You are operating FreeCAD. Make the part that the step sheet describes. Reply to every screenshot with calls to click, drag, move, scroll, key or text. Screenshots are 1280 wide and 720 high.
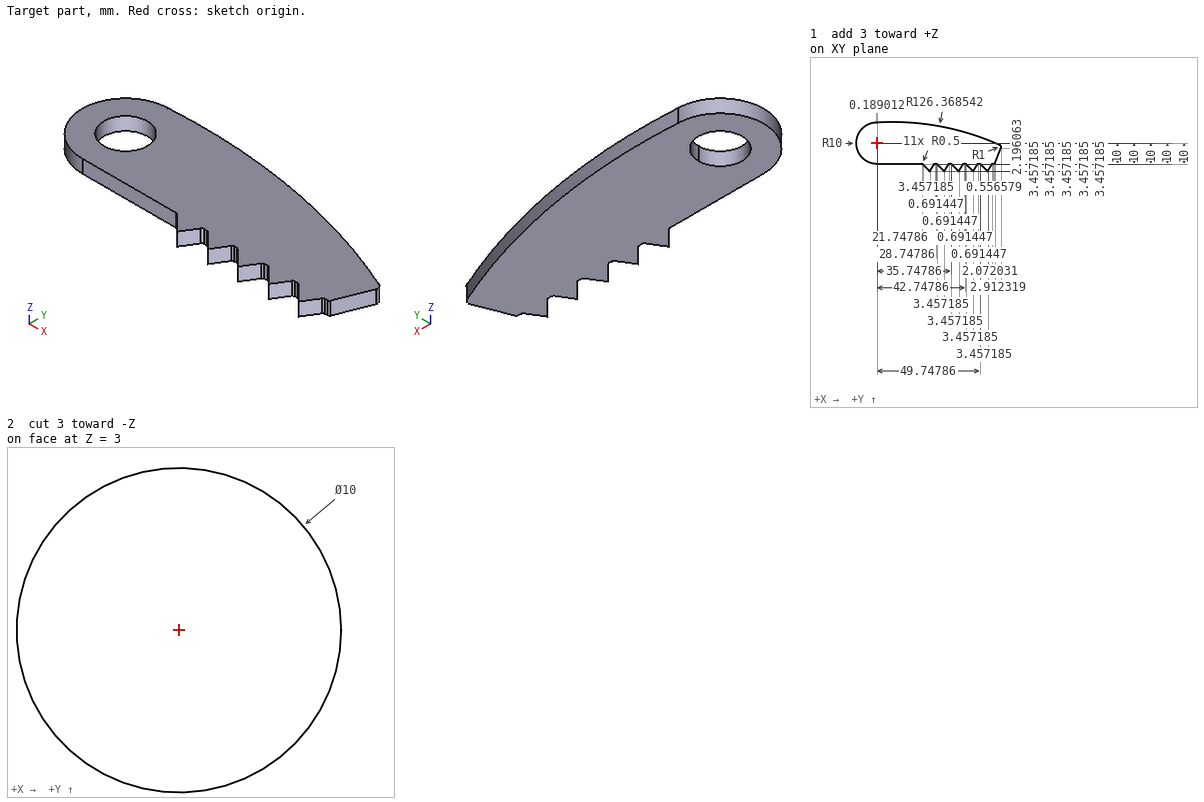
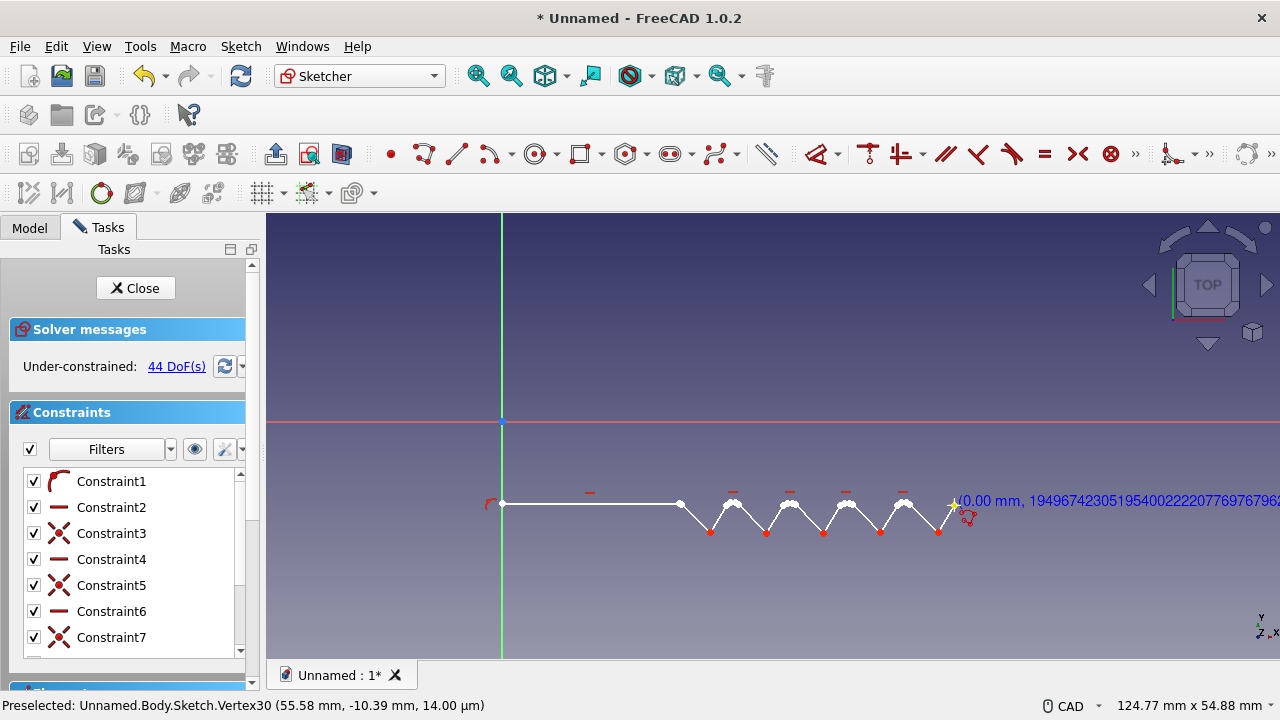
key(g)
key(l)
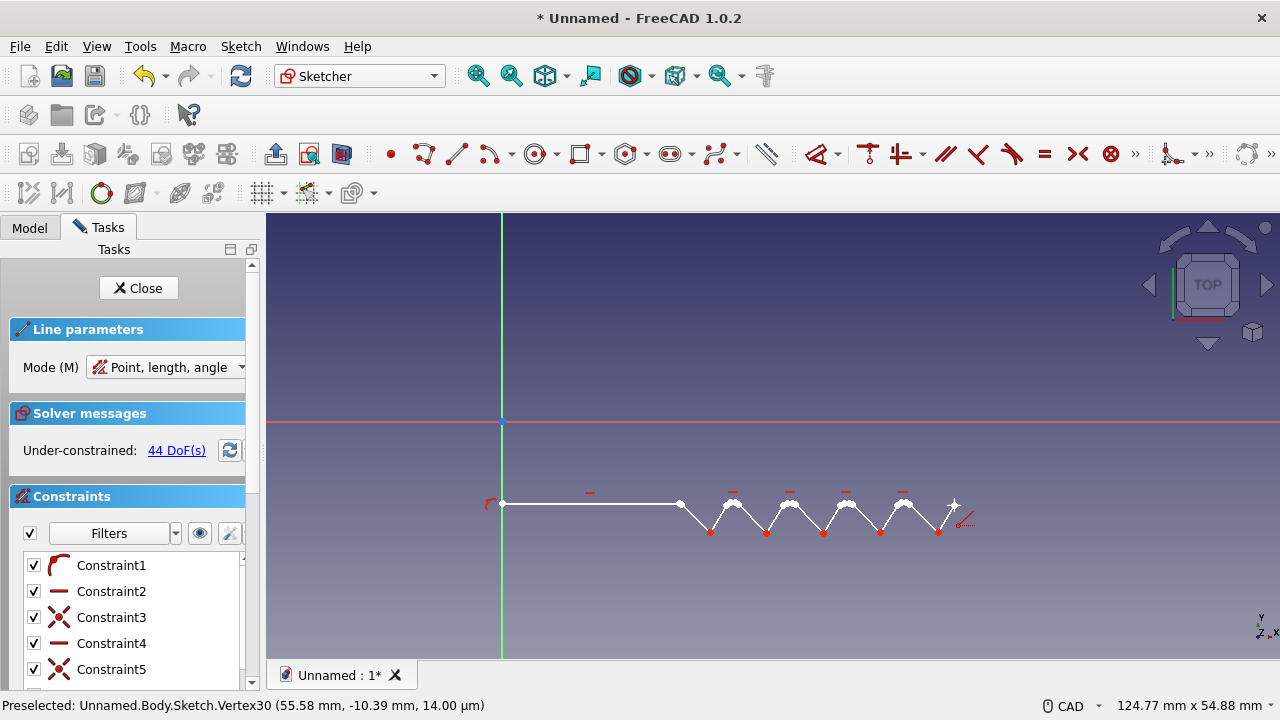
scroll(958, 503, up, 7)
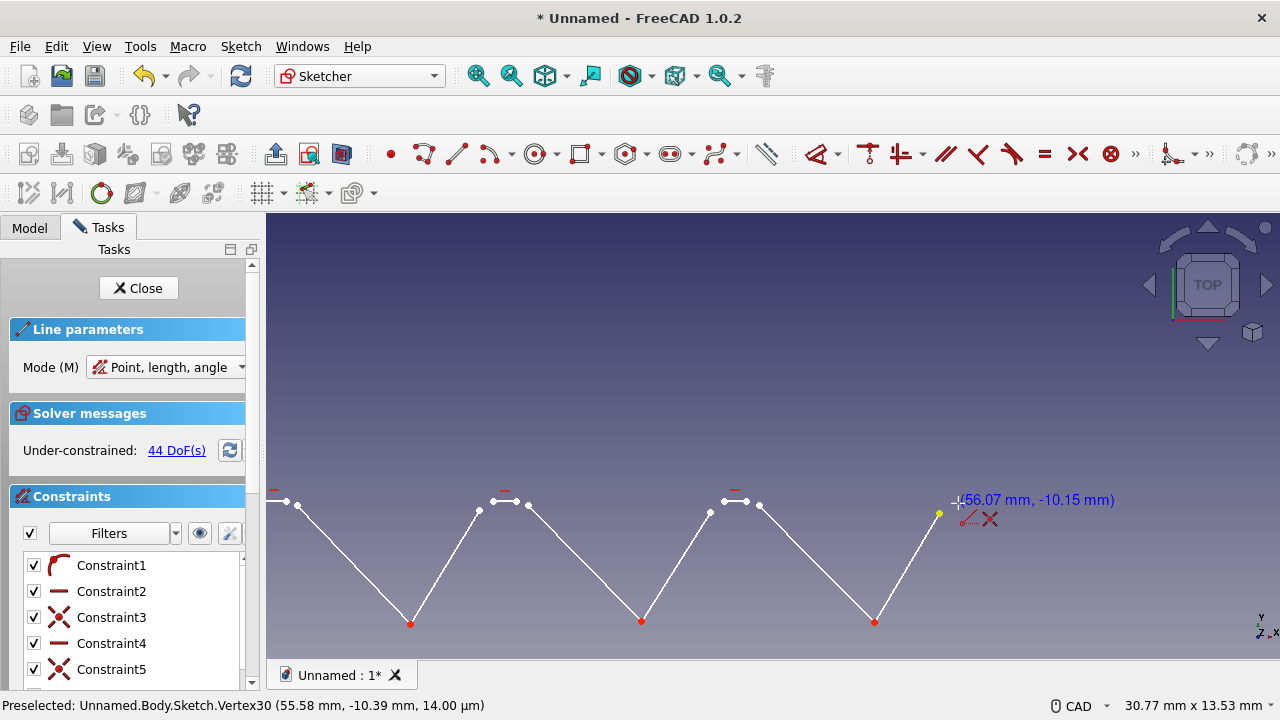
click(955, 500)
click(974, 500)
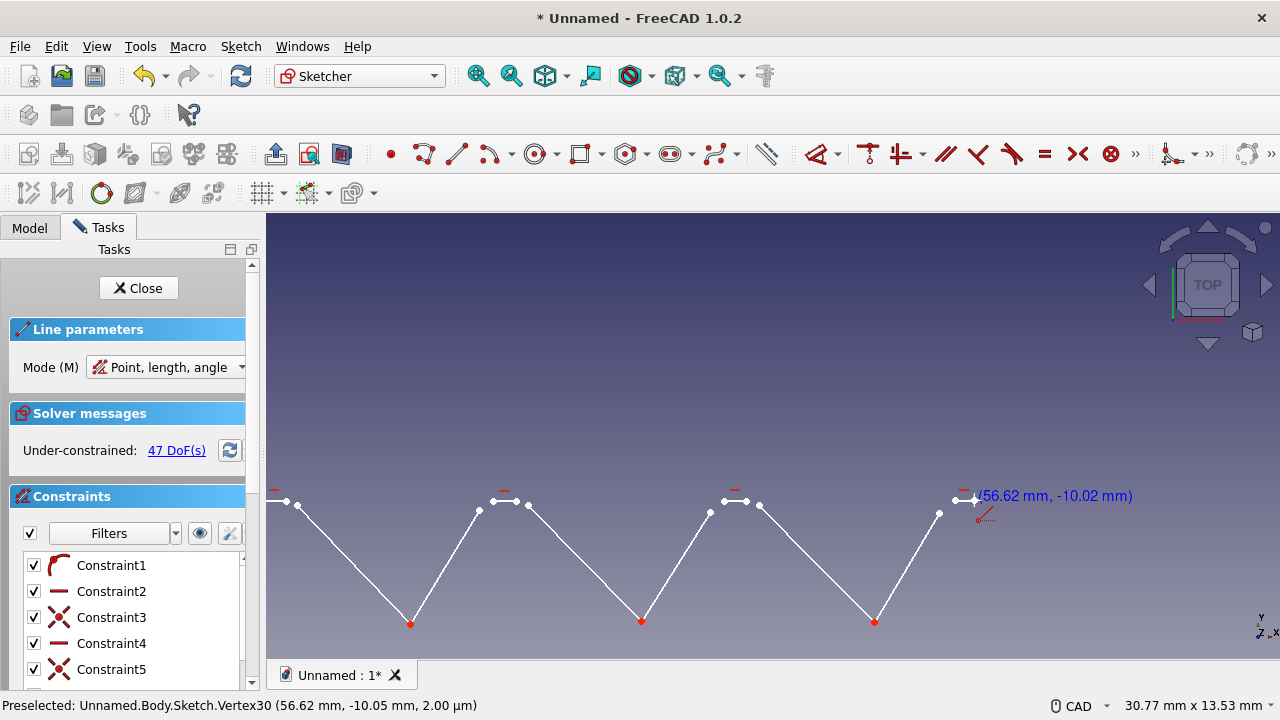
click(989, 490)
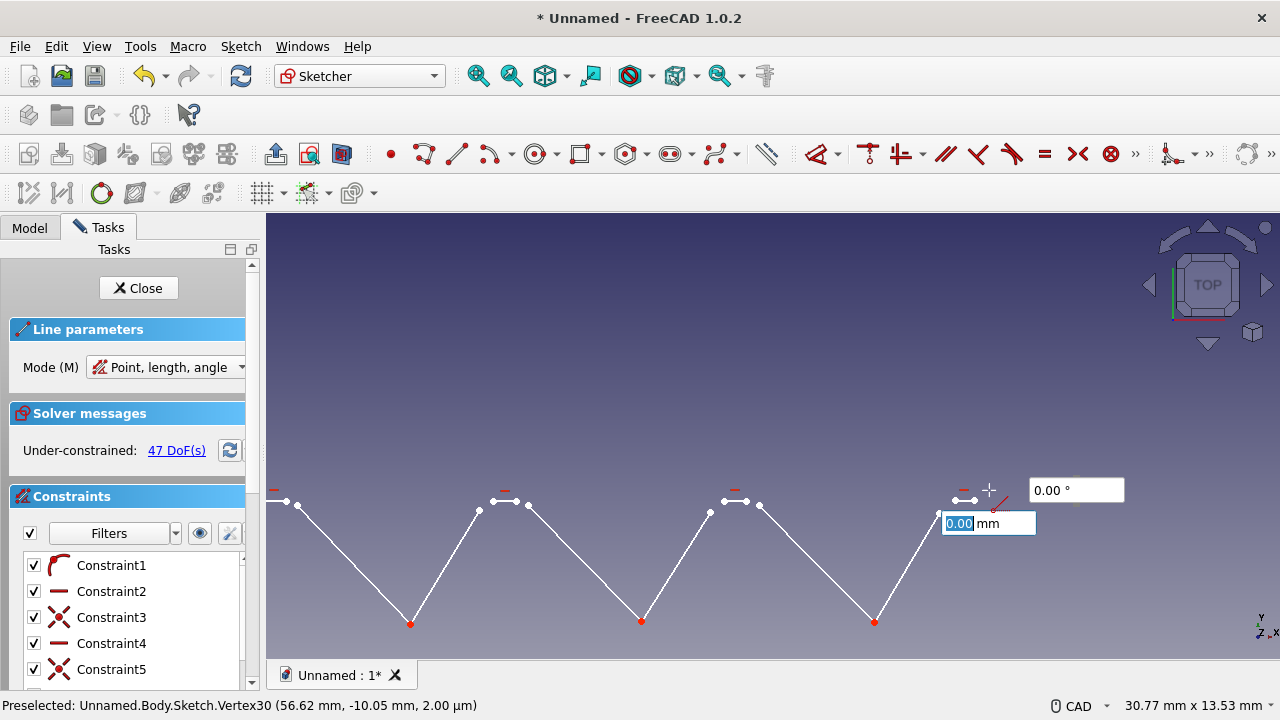
scroll(957, 503, down, 7)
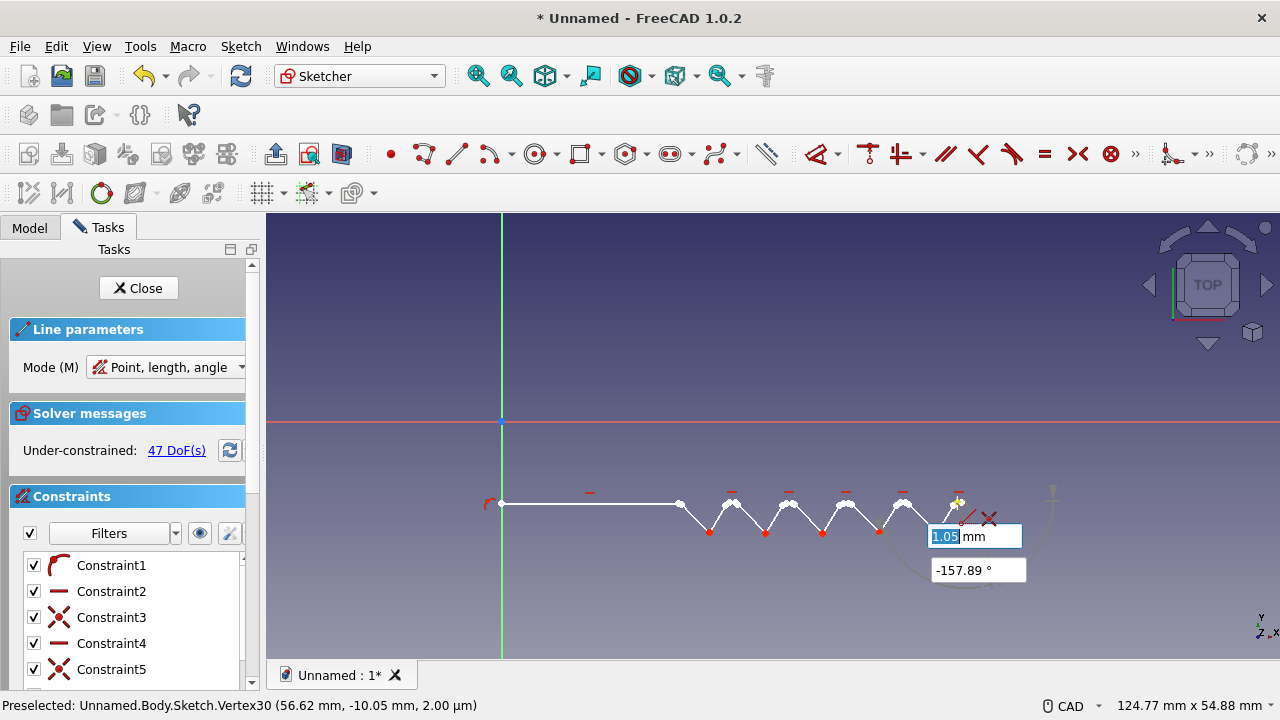
click(989, 439)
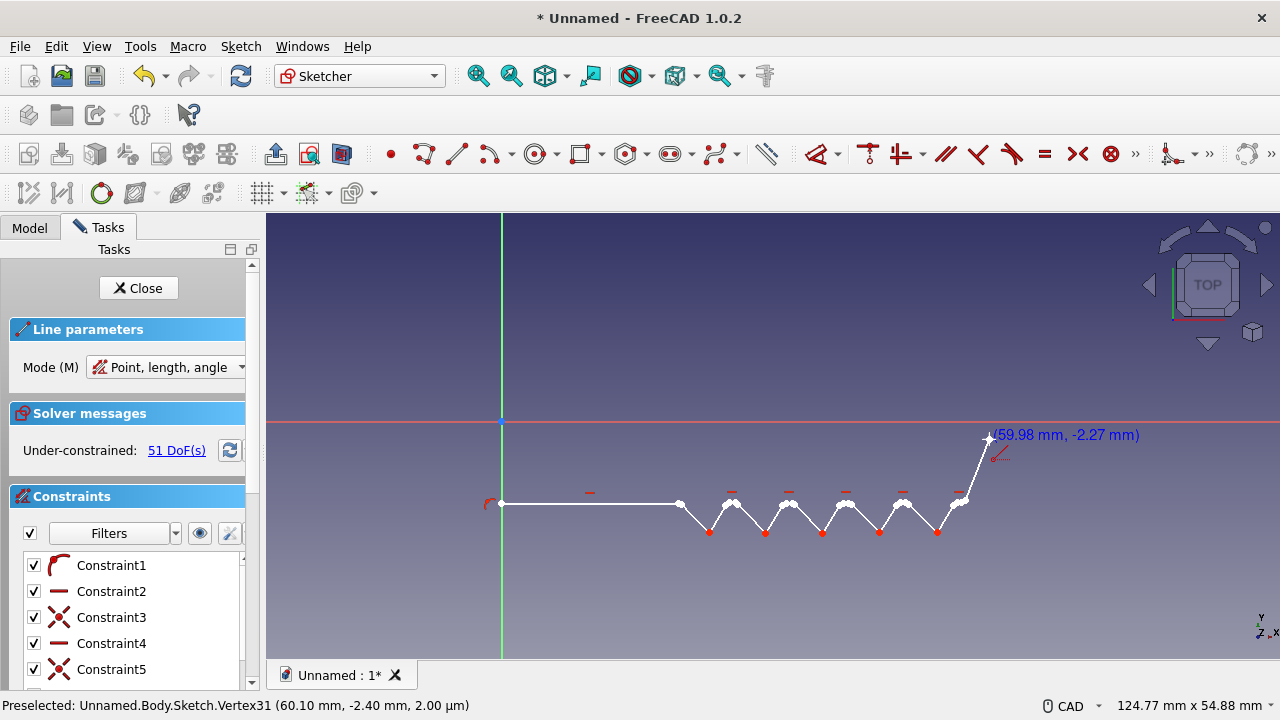
click(512, 154)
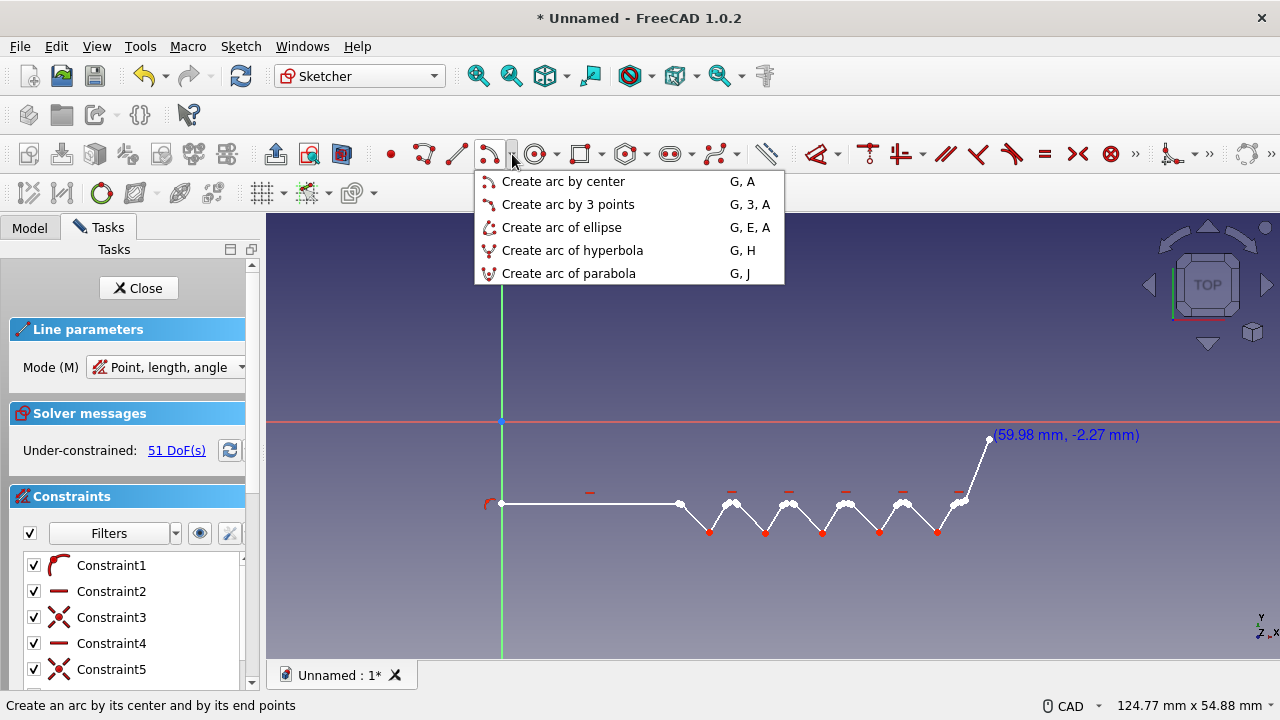
click(630, 204)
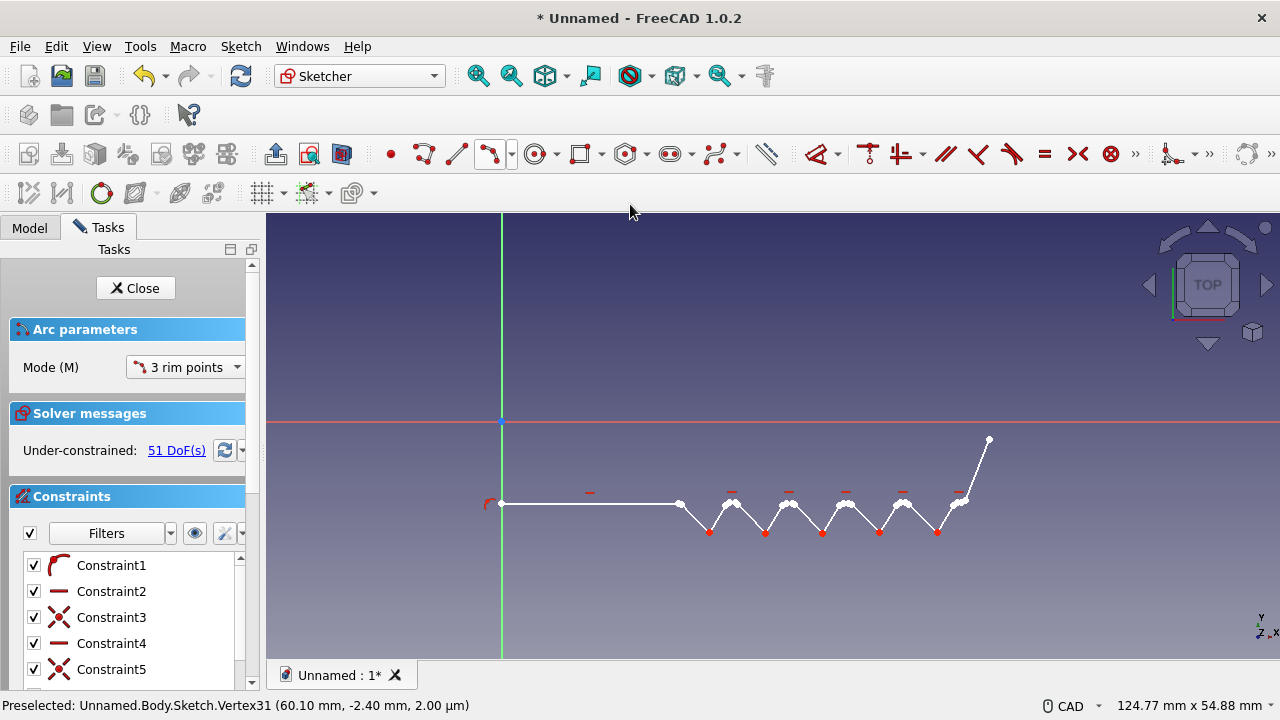
scroll(678, 503, up, 9)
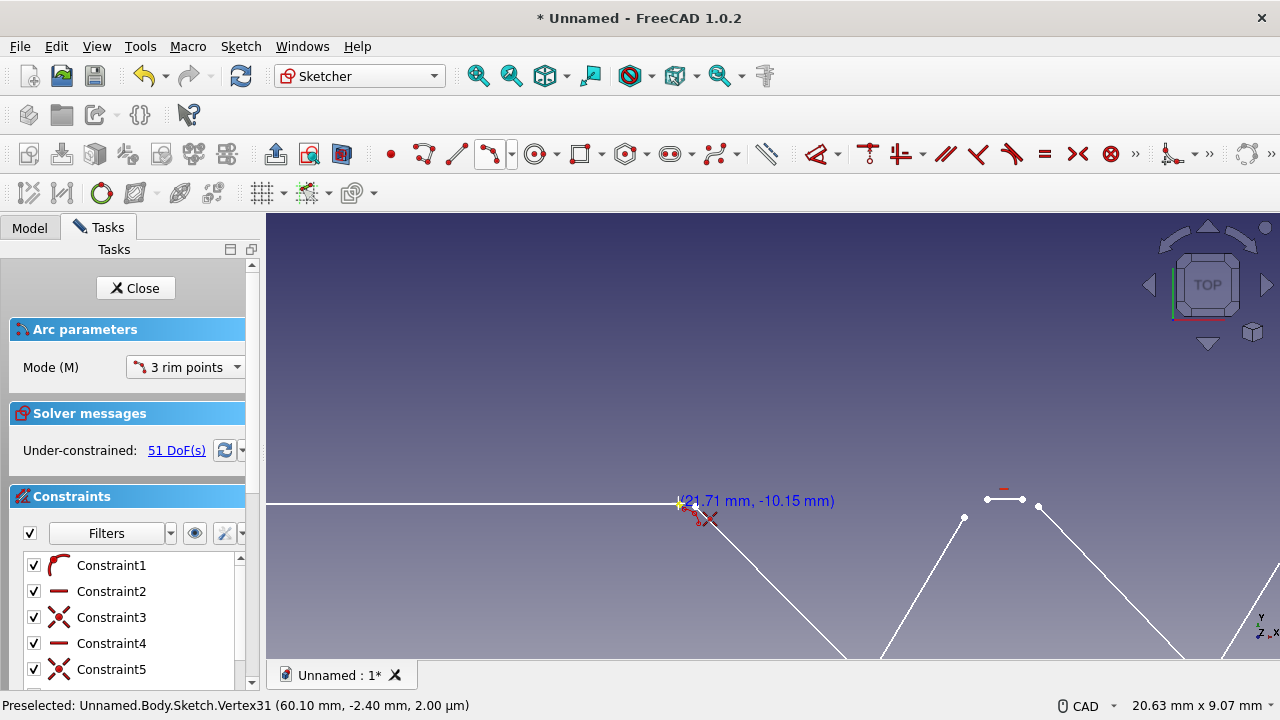
click(679, 504)
click(695, 507)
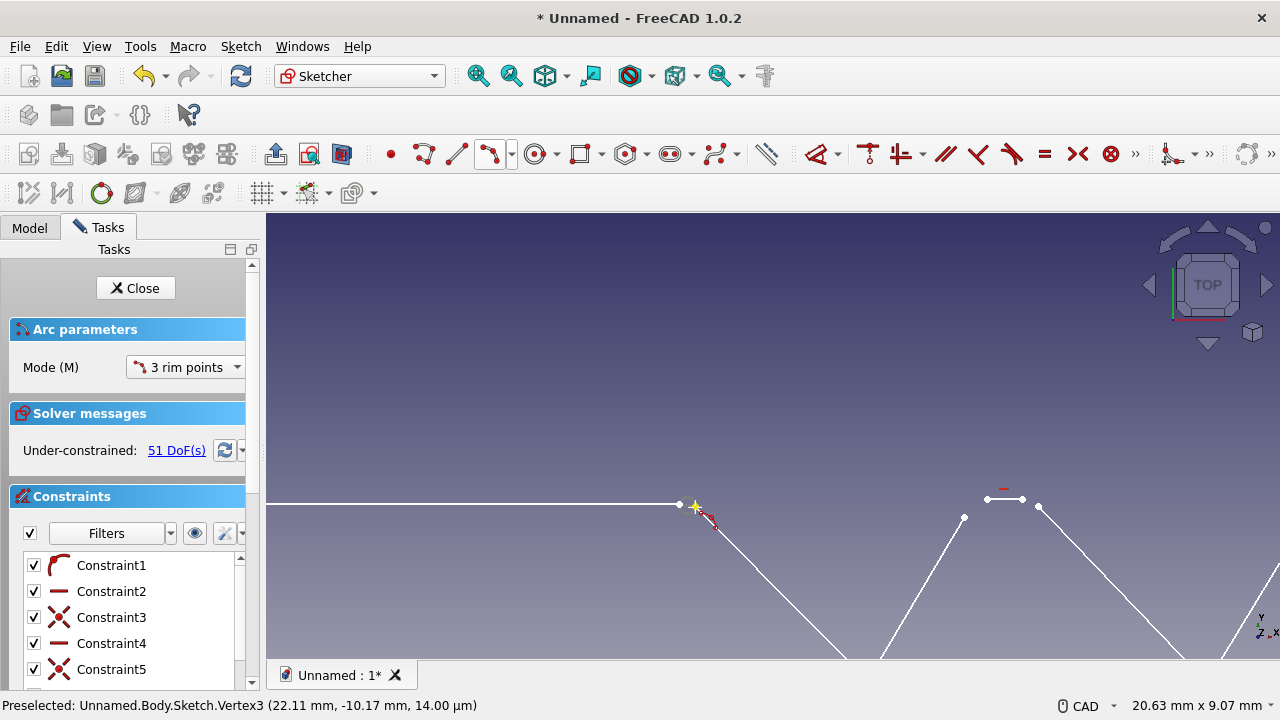
scroll(687, 500, up, 11)